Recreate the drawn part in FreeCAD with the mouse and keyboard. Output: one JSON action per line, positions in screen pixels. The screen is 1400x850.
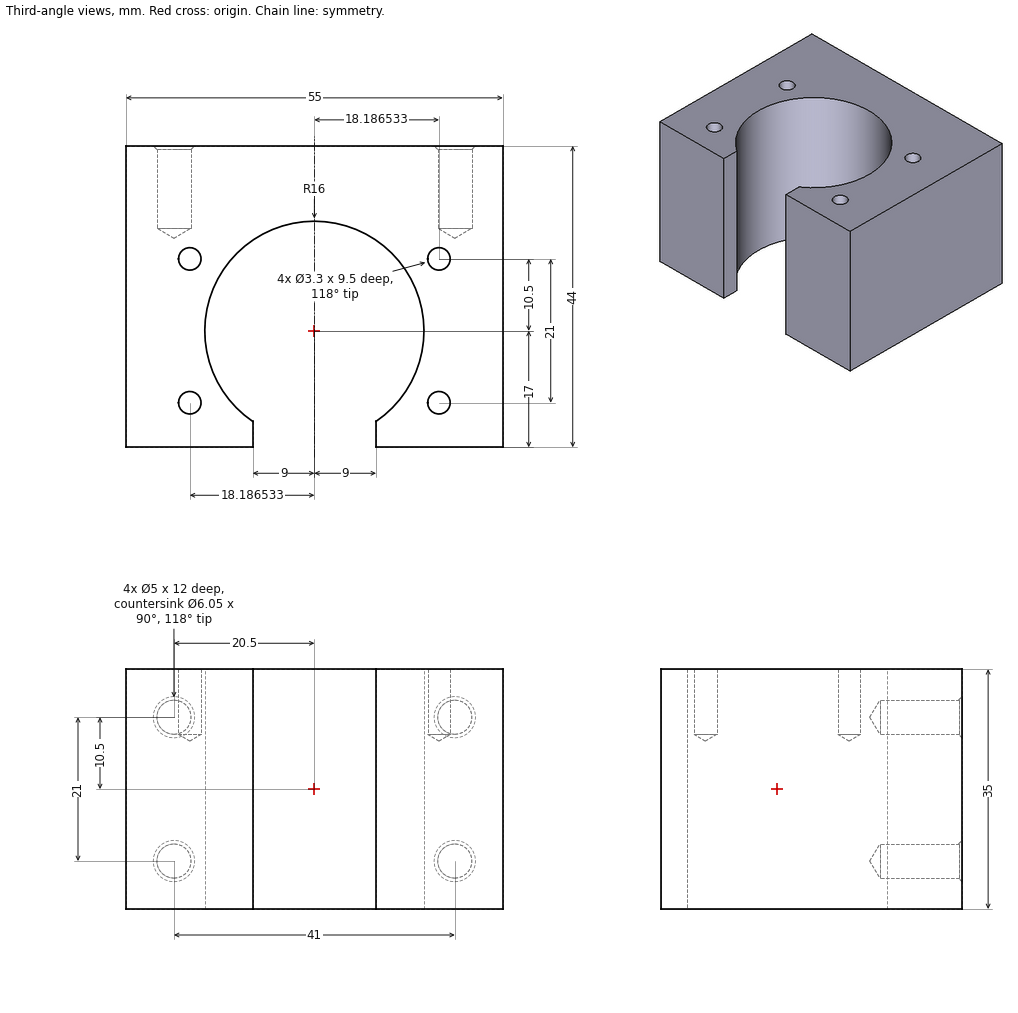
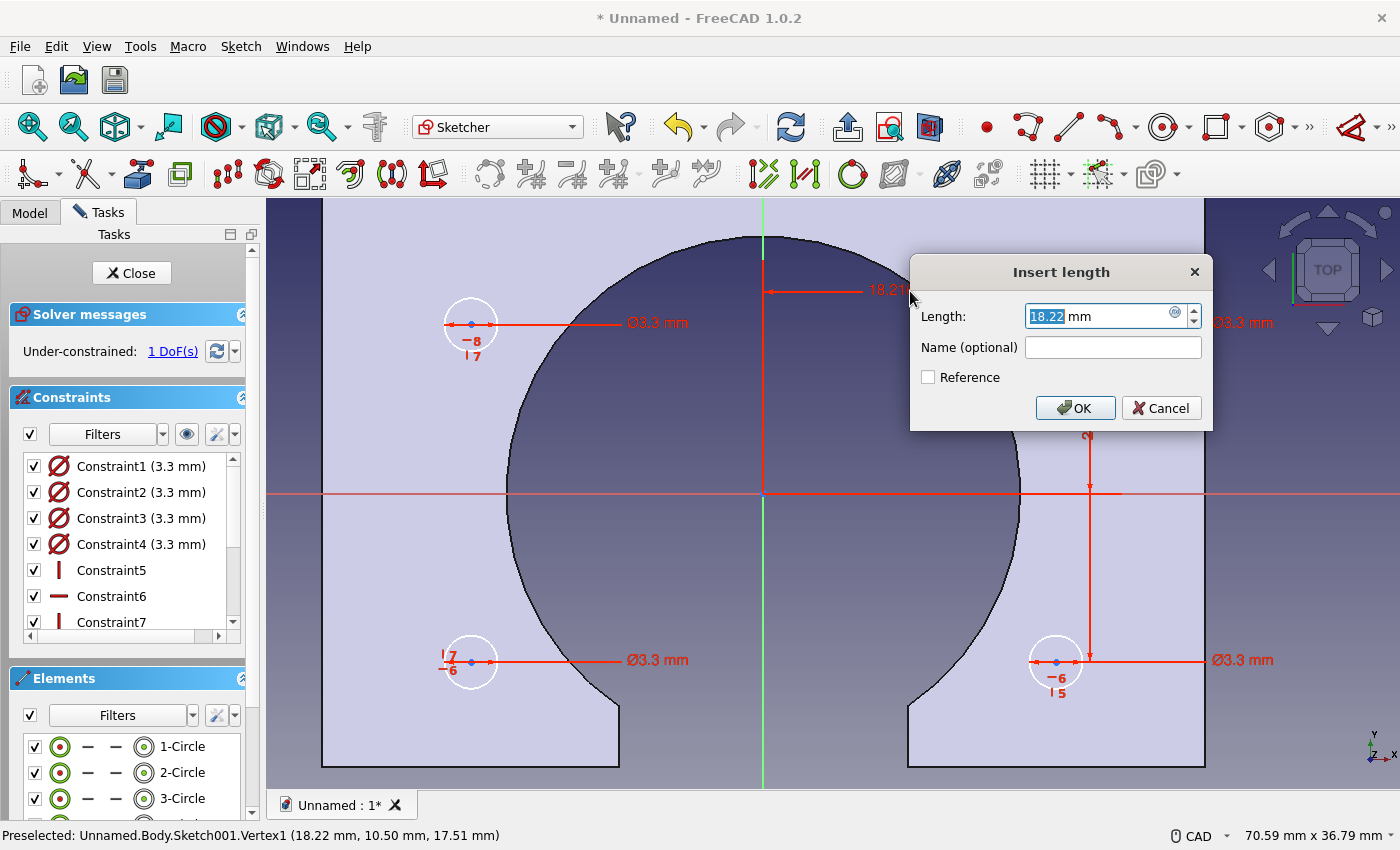
{"action": "type", "text": "18.186533"}
{"action": "key", "text": "Return"}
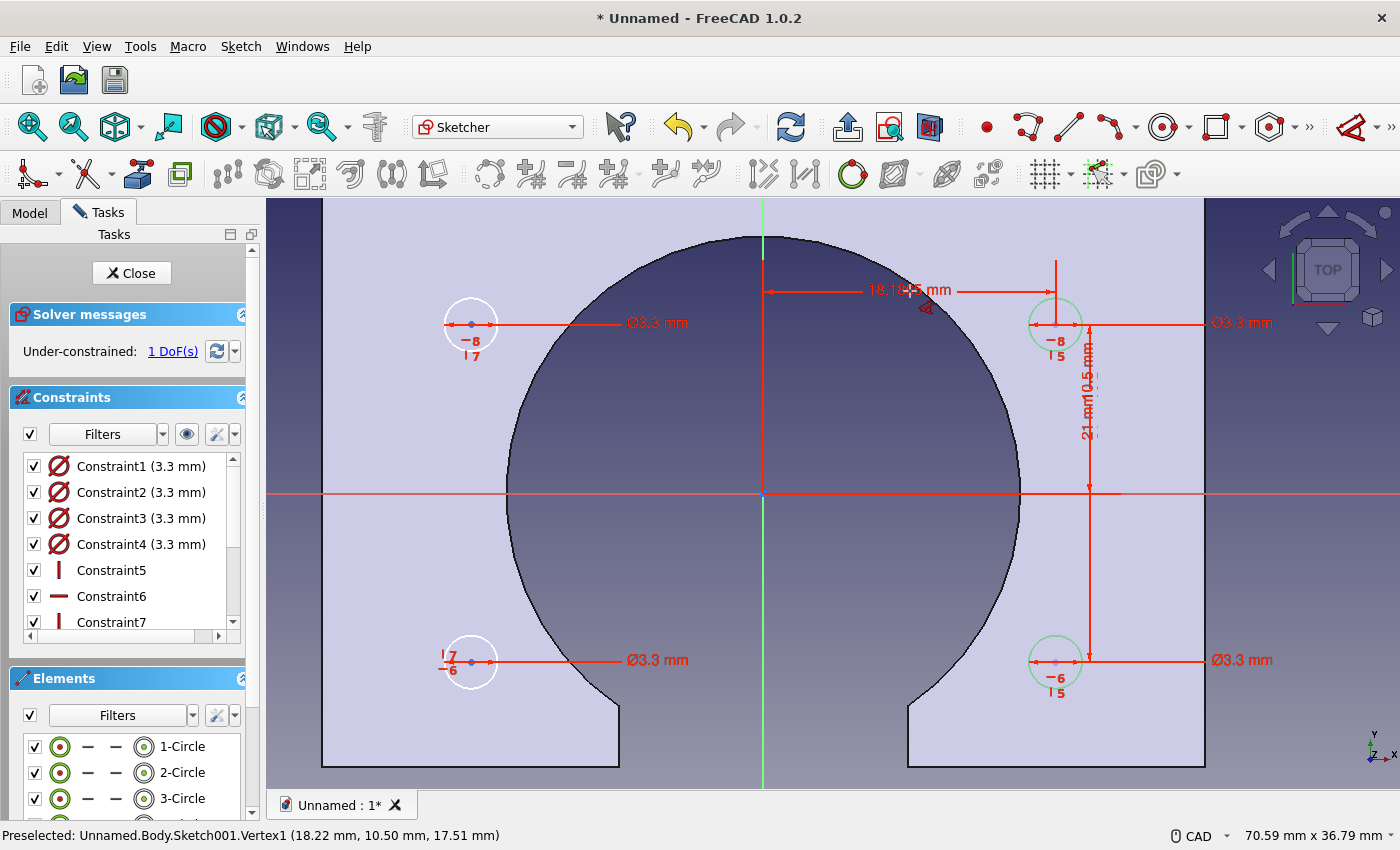
{"action": "left_click", "coordinate": [471, 662]}
{"action": "left_click", "coordinate": [617, 696]}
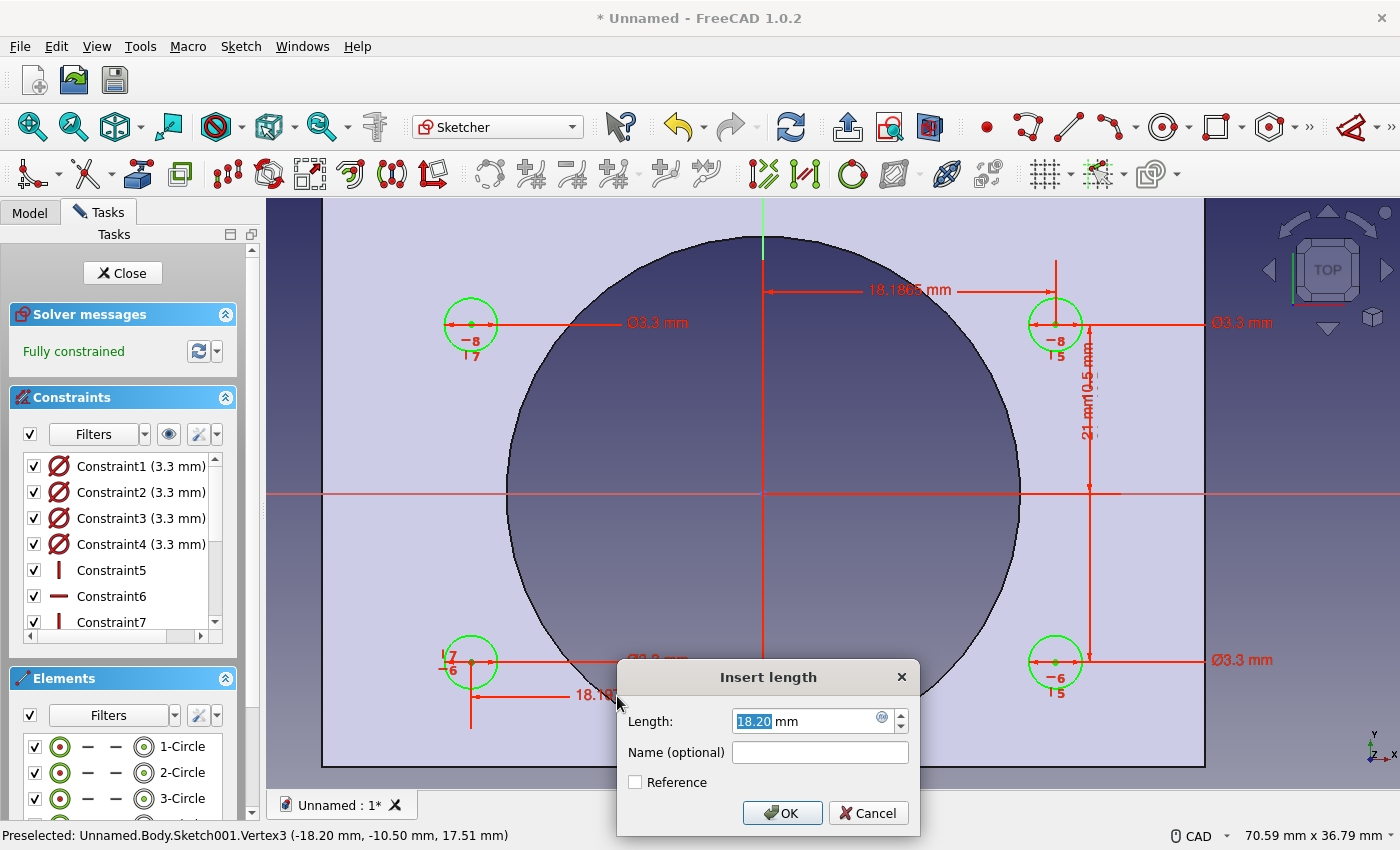
{"action": "type", "text": "18.186533"}
{"action": "key", "text": "Return"}
{"action": "key", "text": "Escape"}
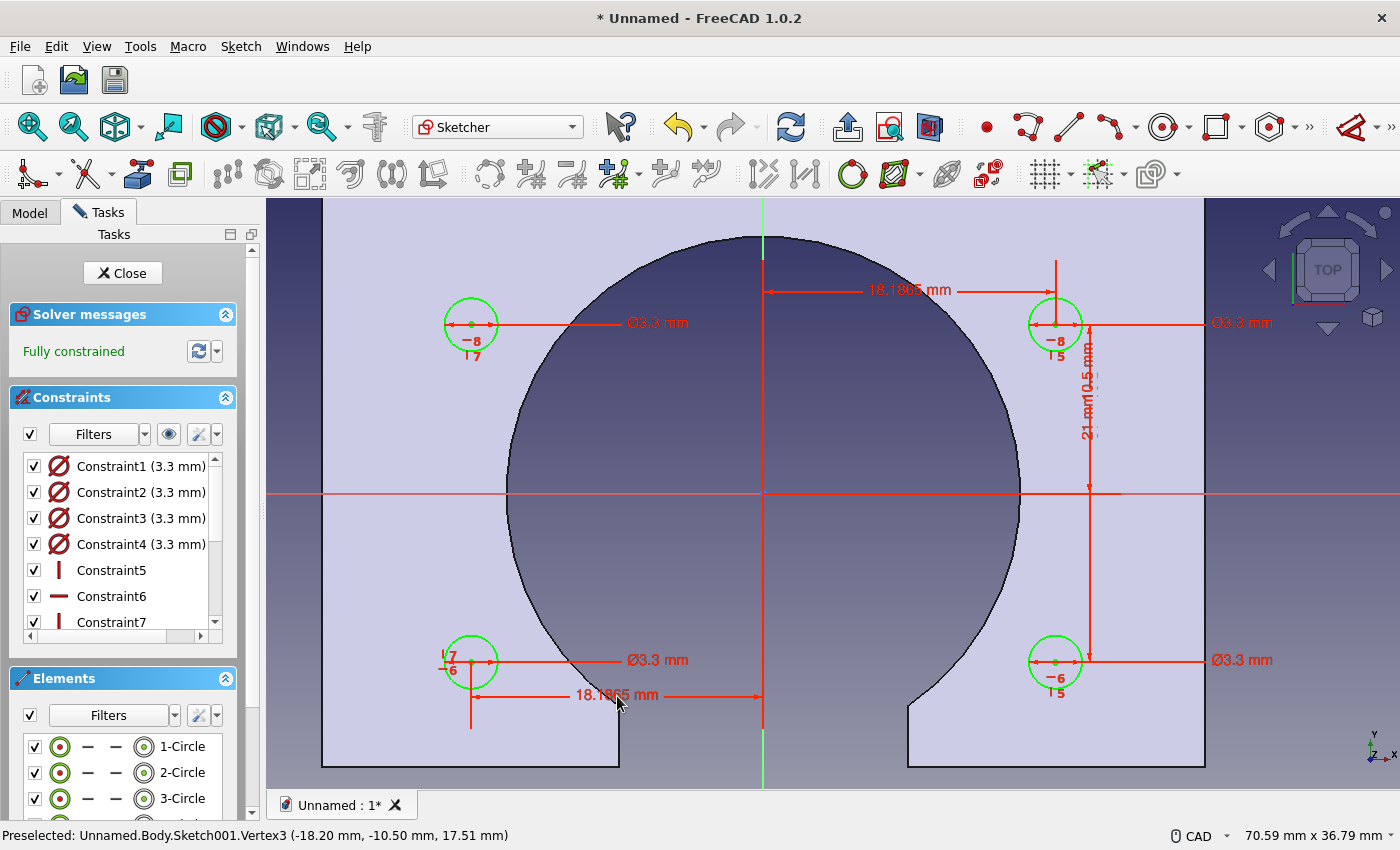
{"action": "left_click", "coordinate": [123, 273]}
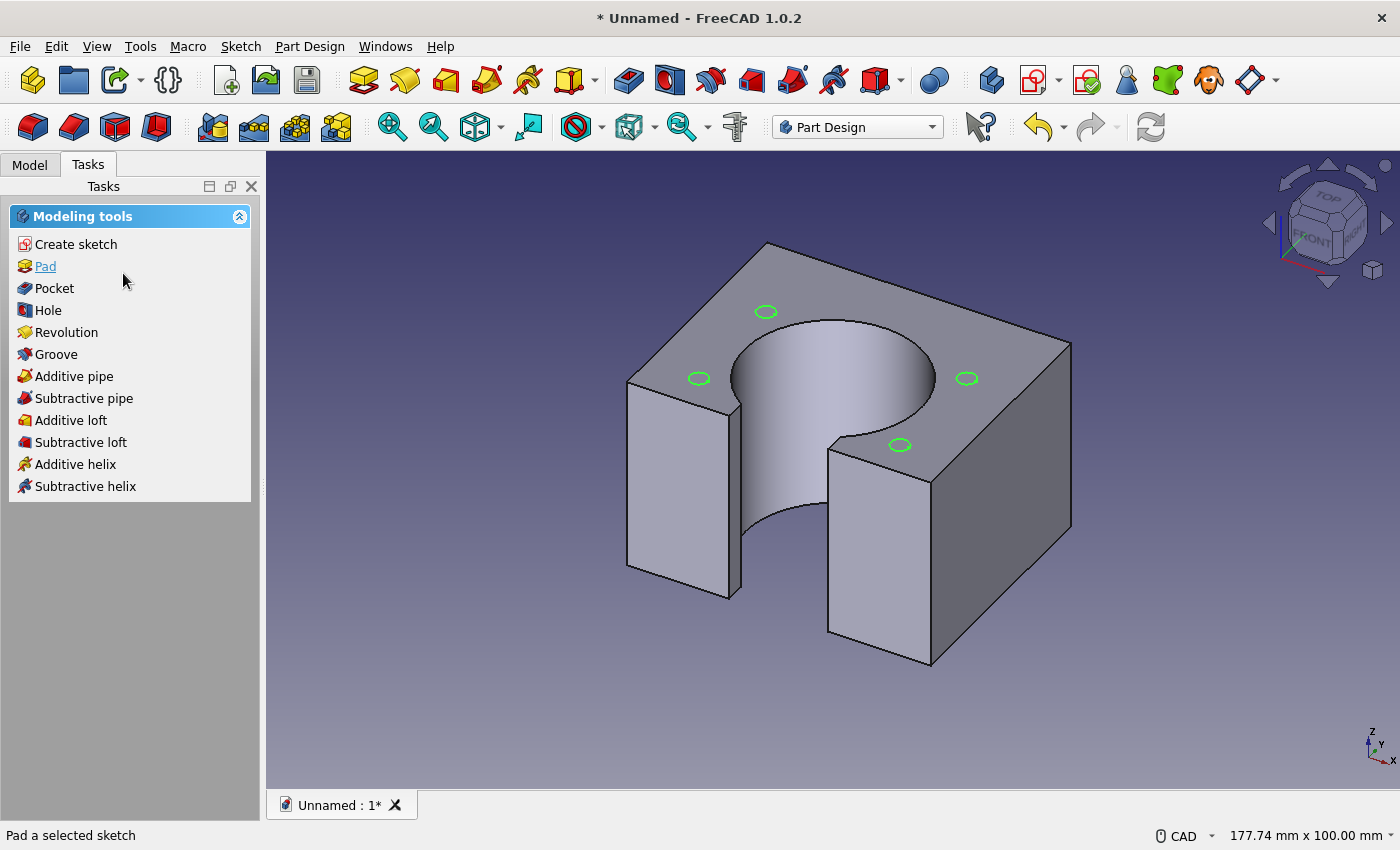
{"action": "left_click", "coordinate": [670, 80]}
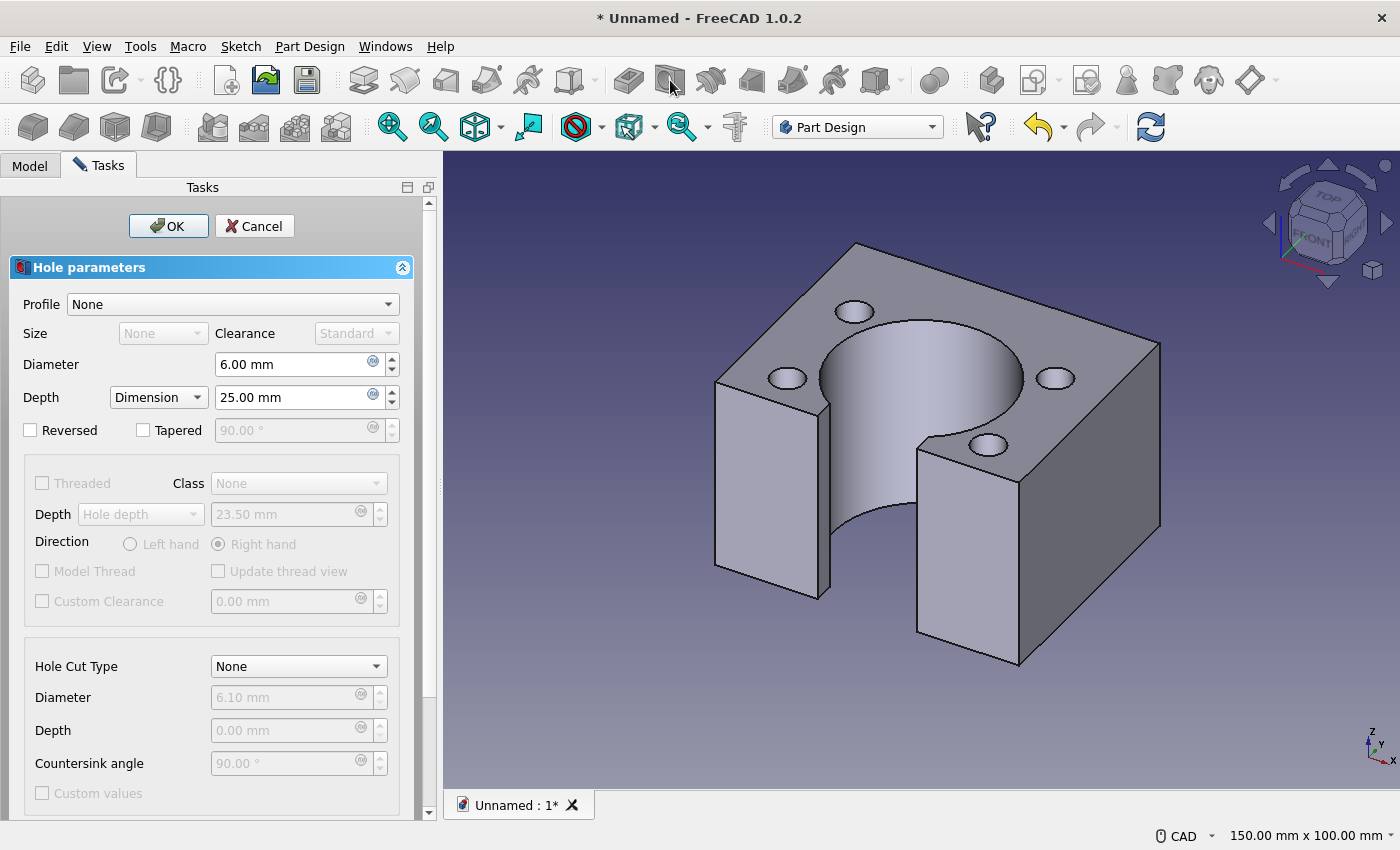
{"action": "triple_click", "coordinate": [300, 364]}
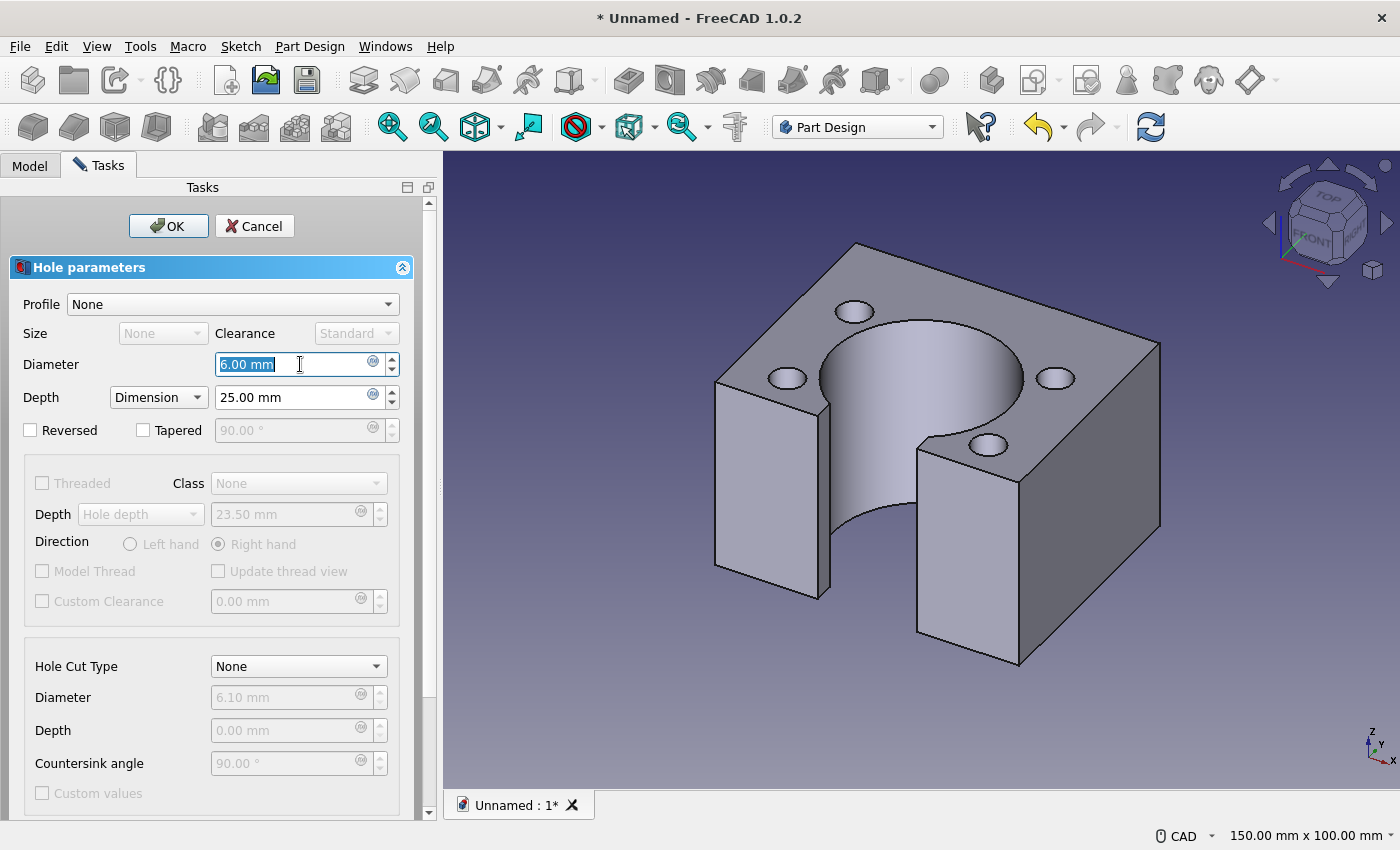
{"action": "type", "text": "3.3"}
{"action": "key", "text": "Tab"}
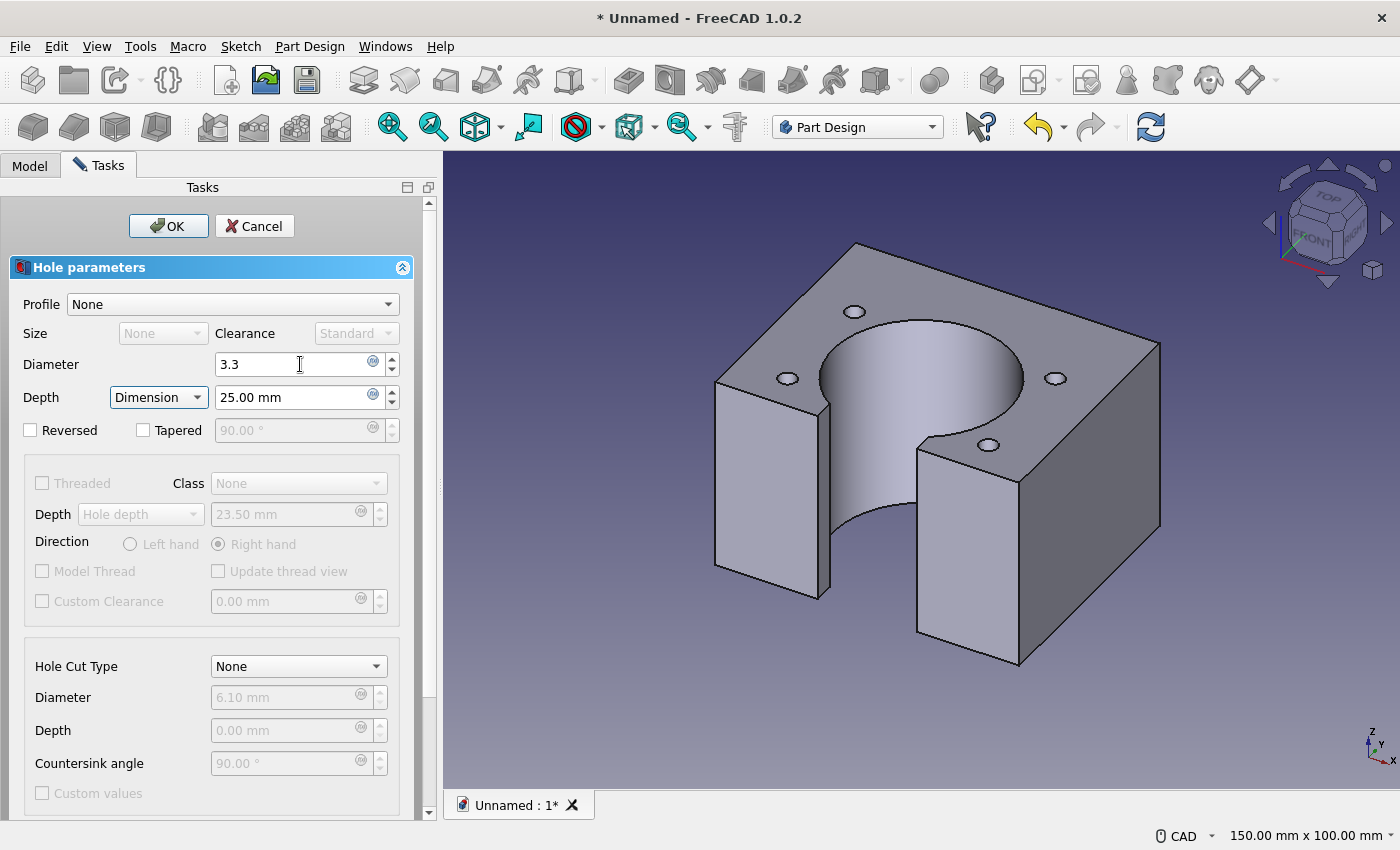
{"action": "triple_click", "coordinate": [300, 398]}